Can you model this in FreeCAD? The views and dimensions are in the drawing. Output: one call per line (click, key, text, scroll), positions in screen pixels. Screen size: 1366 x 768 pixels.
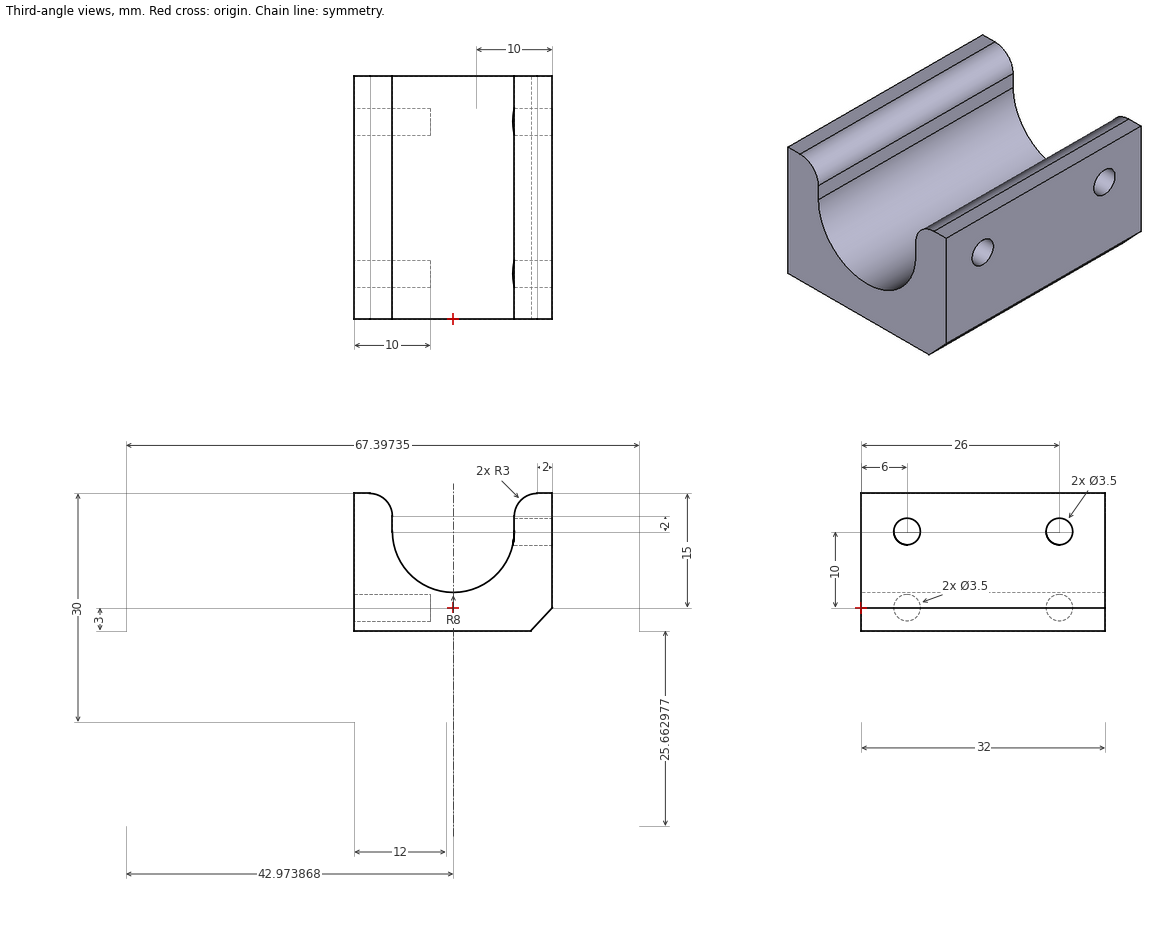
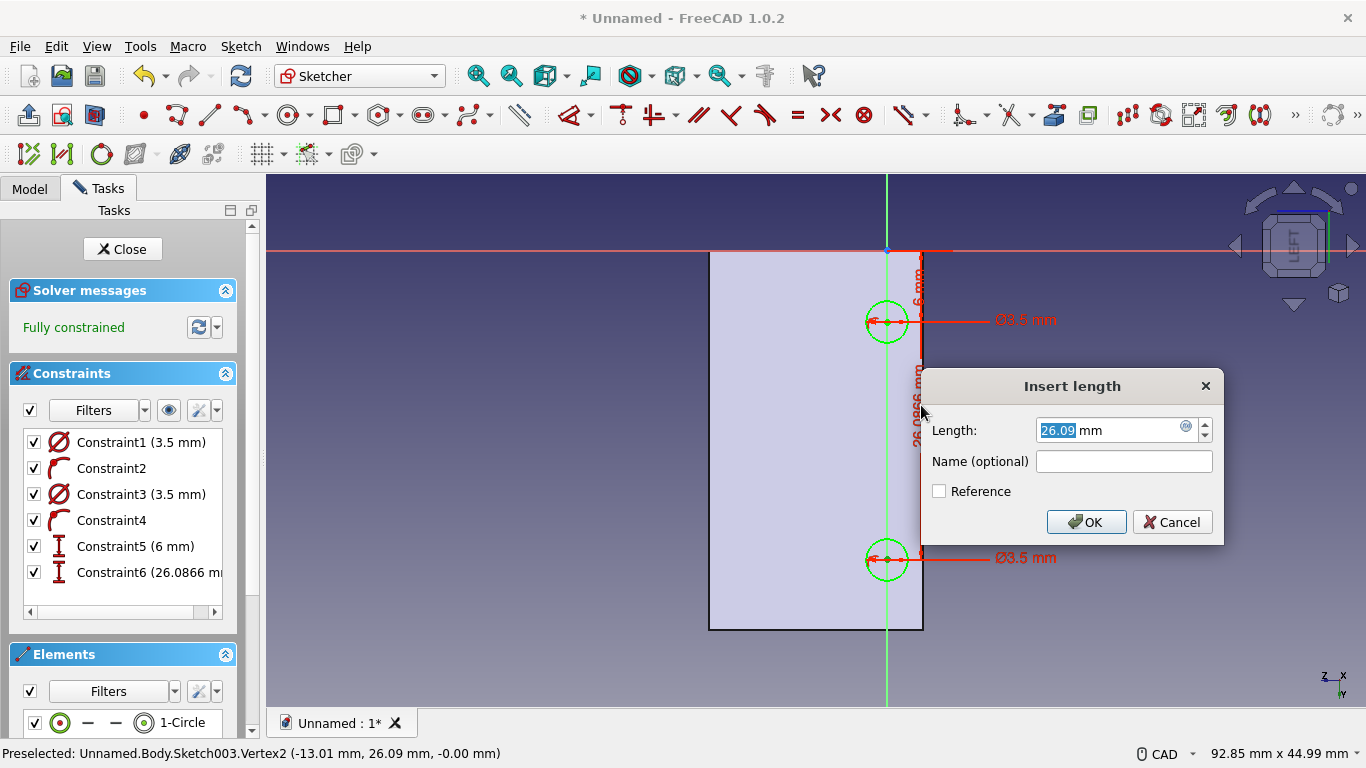
text(26)
key(Return)
key(Escape)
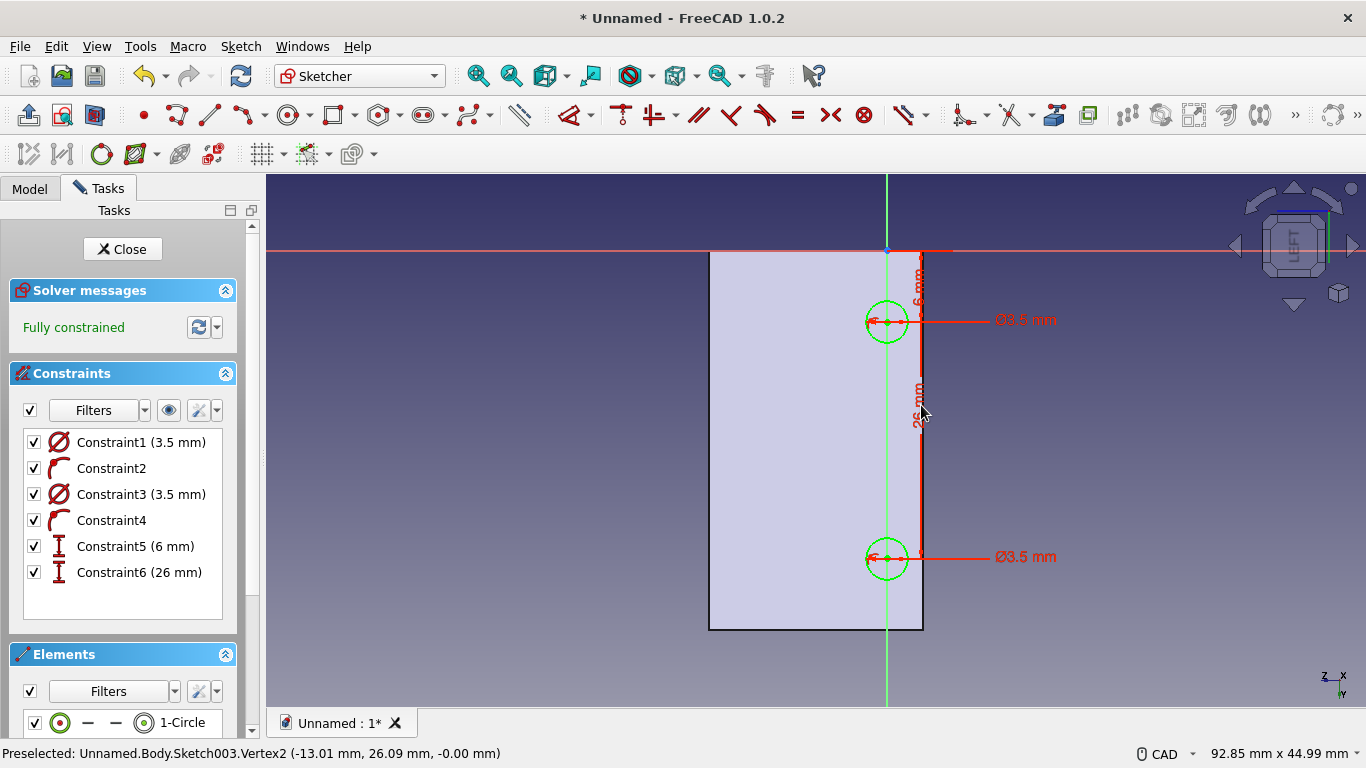
click(123, 249)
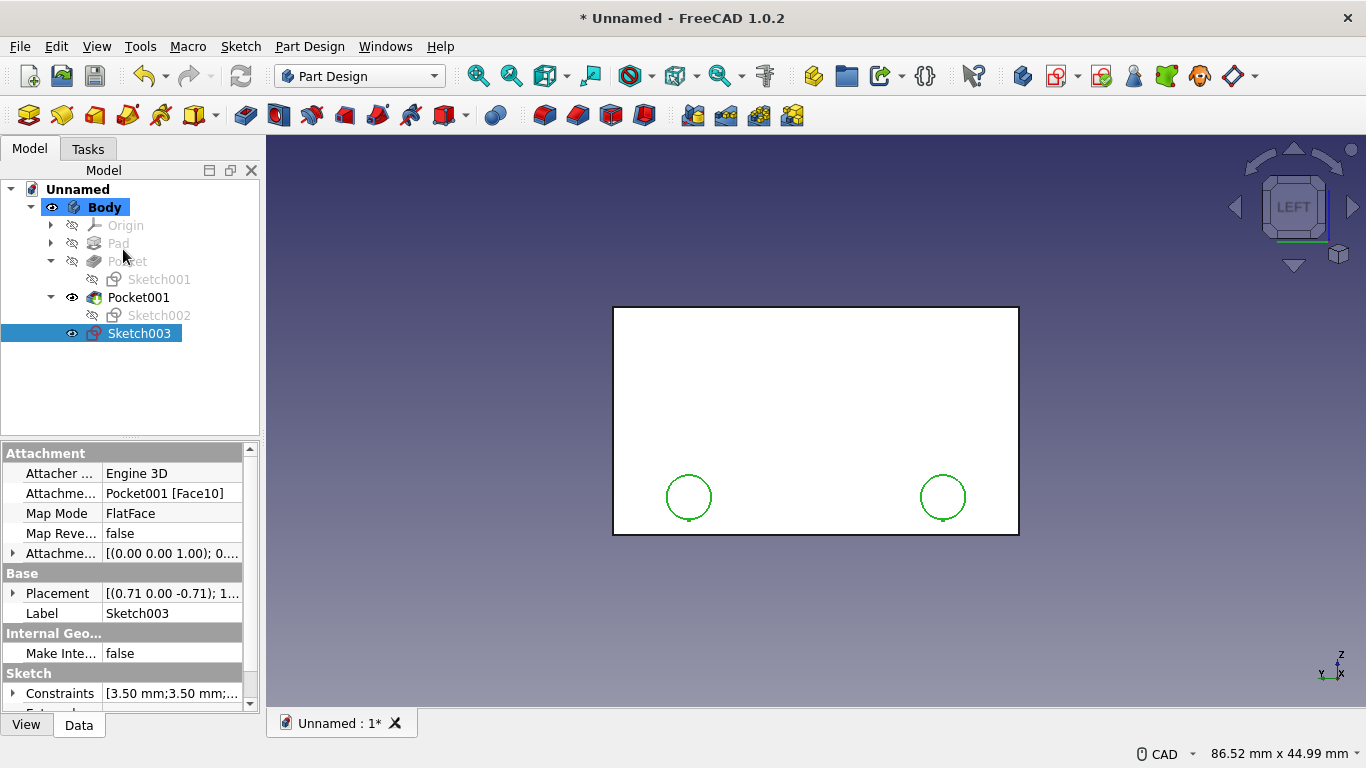
click(246, 116)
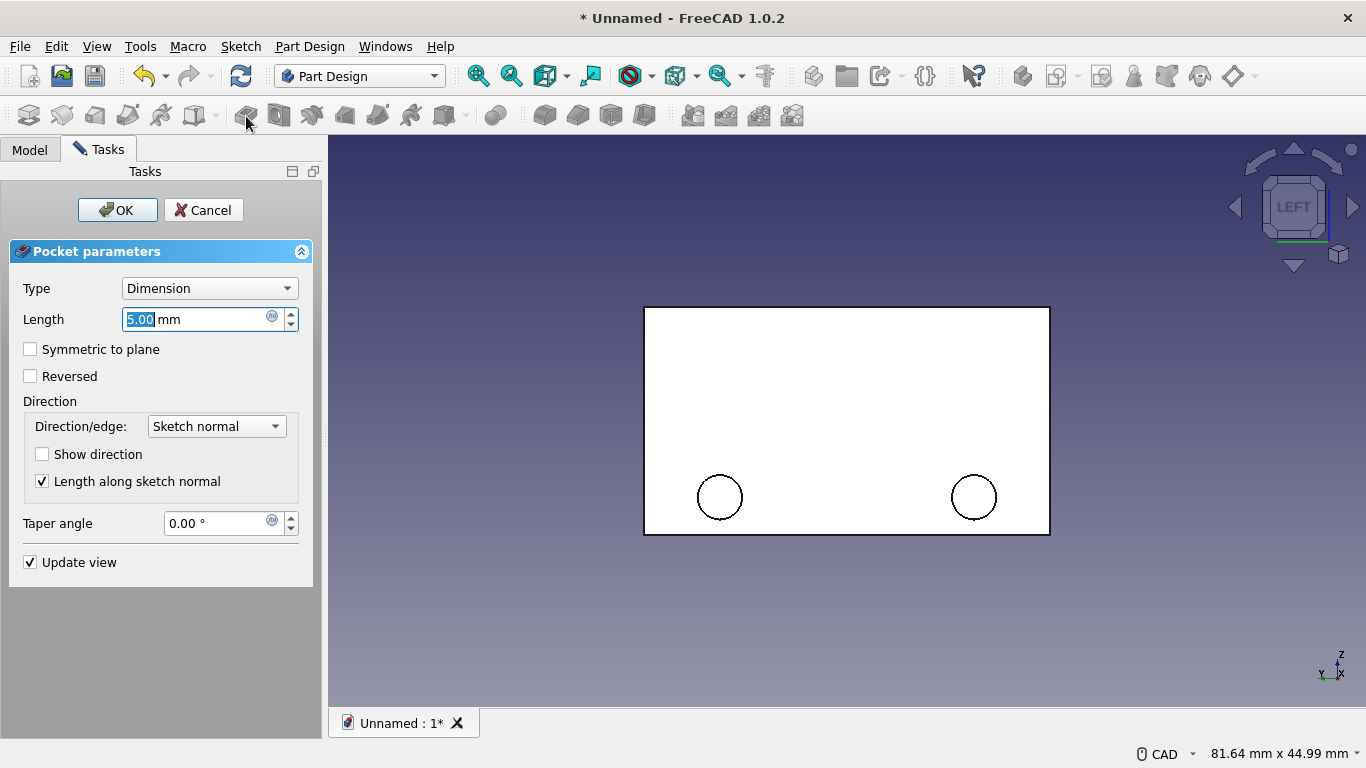
text(10)
key(Tab)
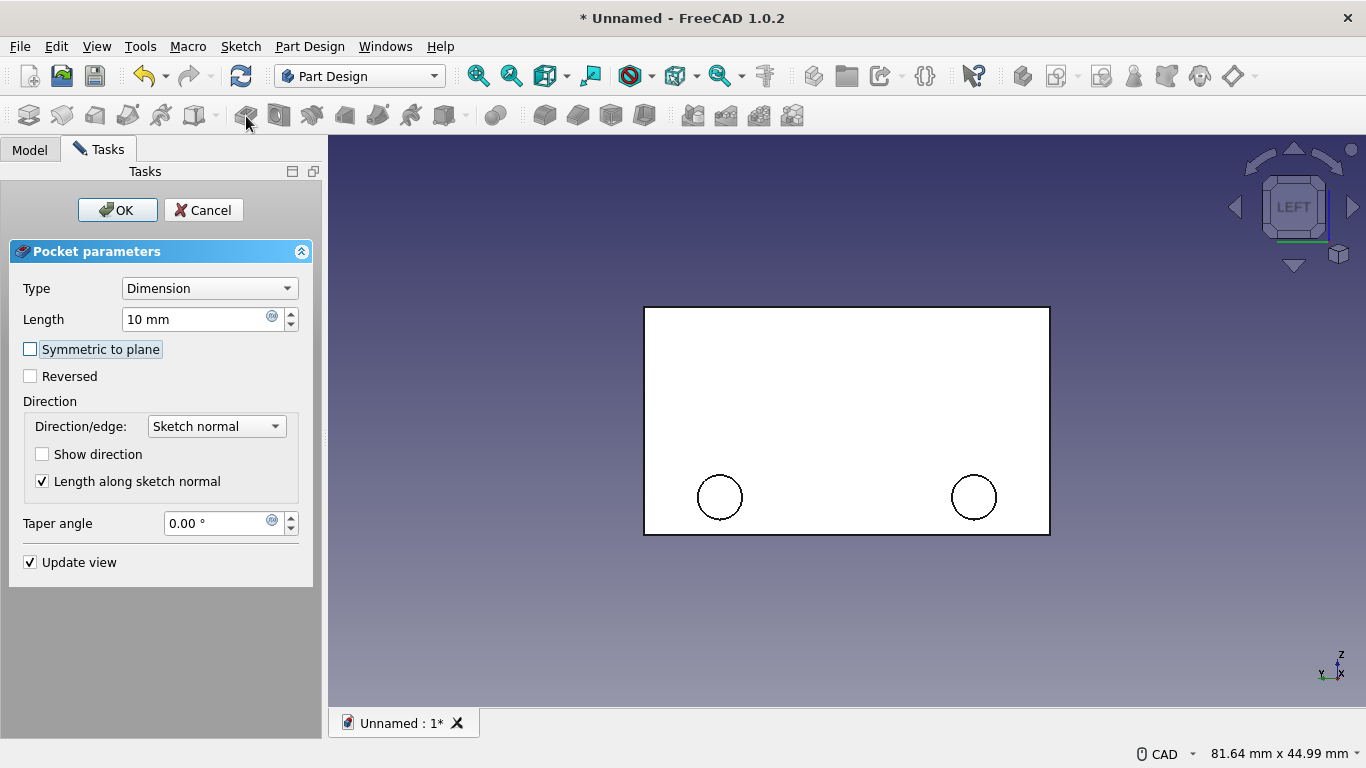
click(118, 210)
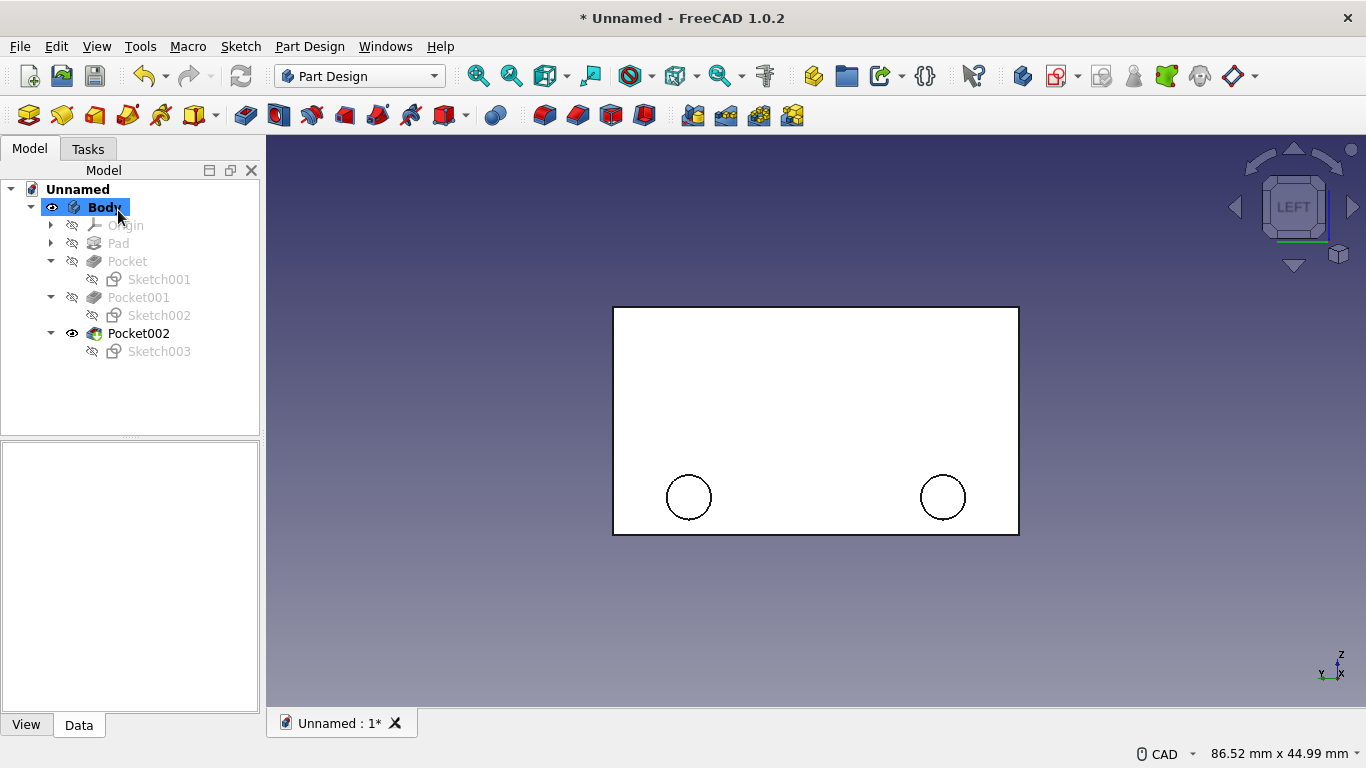
key(0)